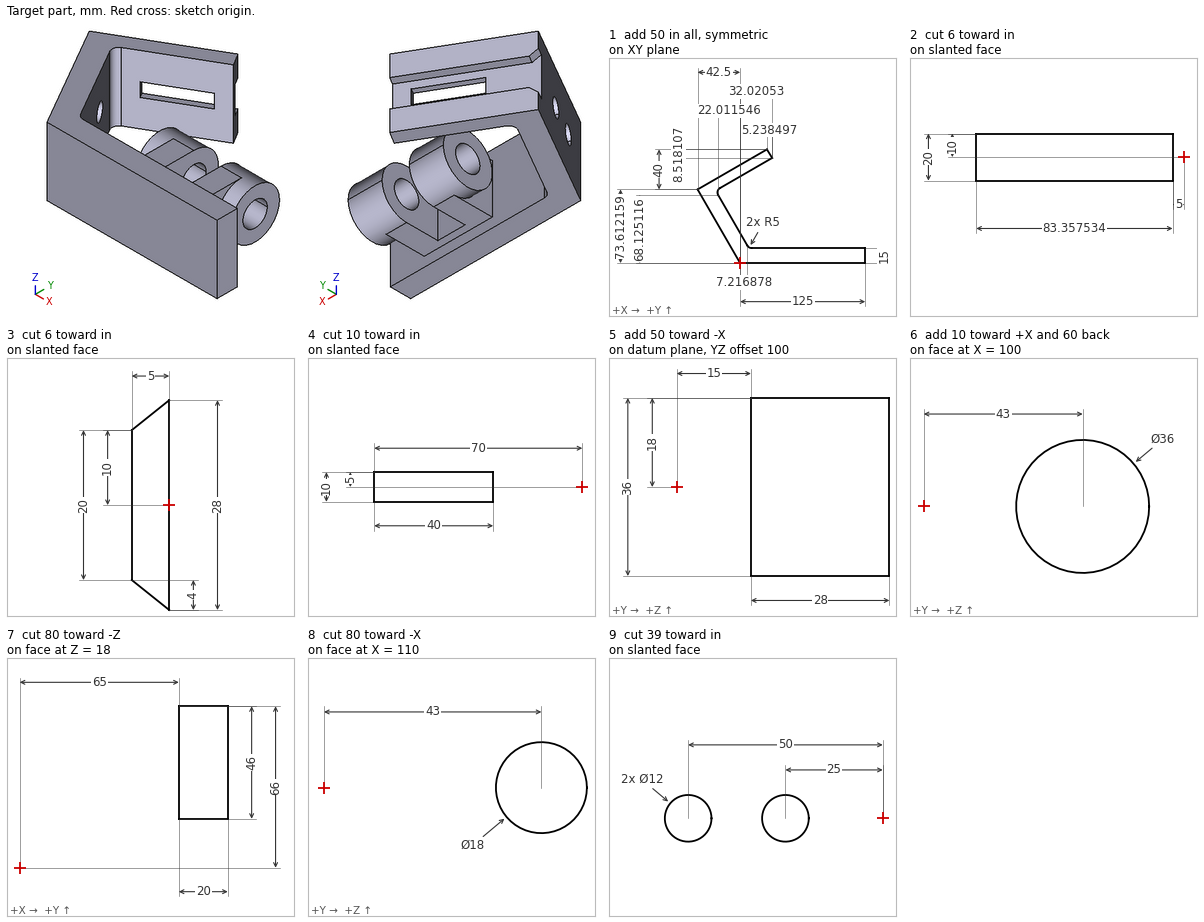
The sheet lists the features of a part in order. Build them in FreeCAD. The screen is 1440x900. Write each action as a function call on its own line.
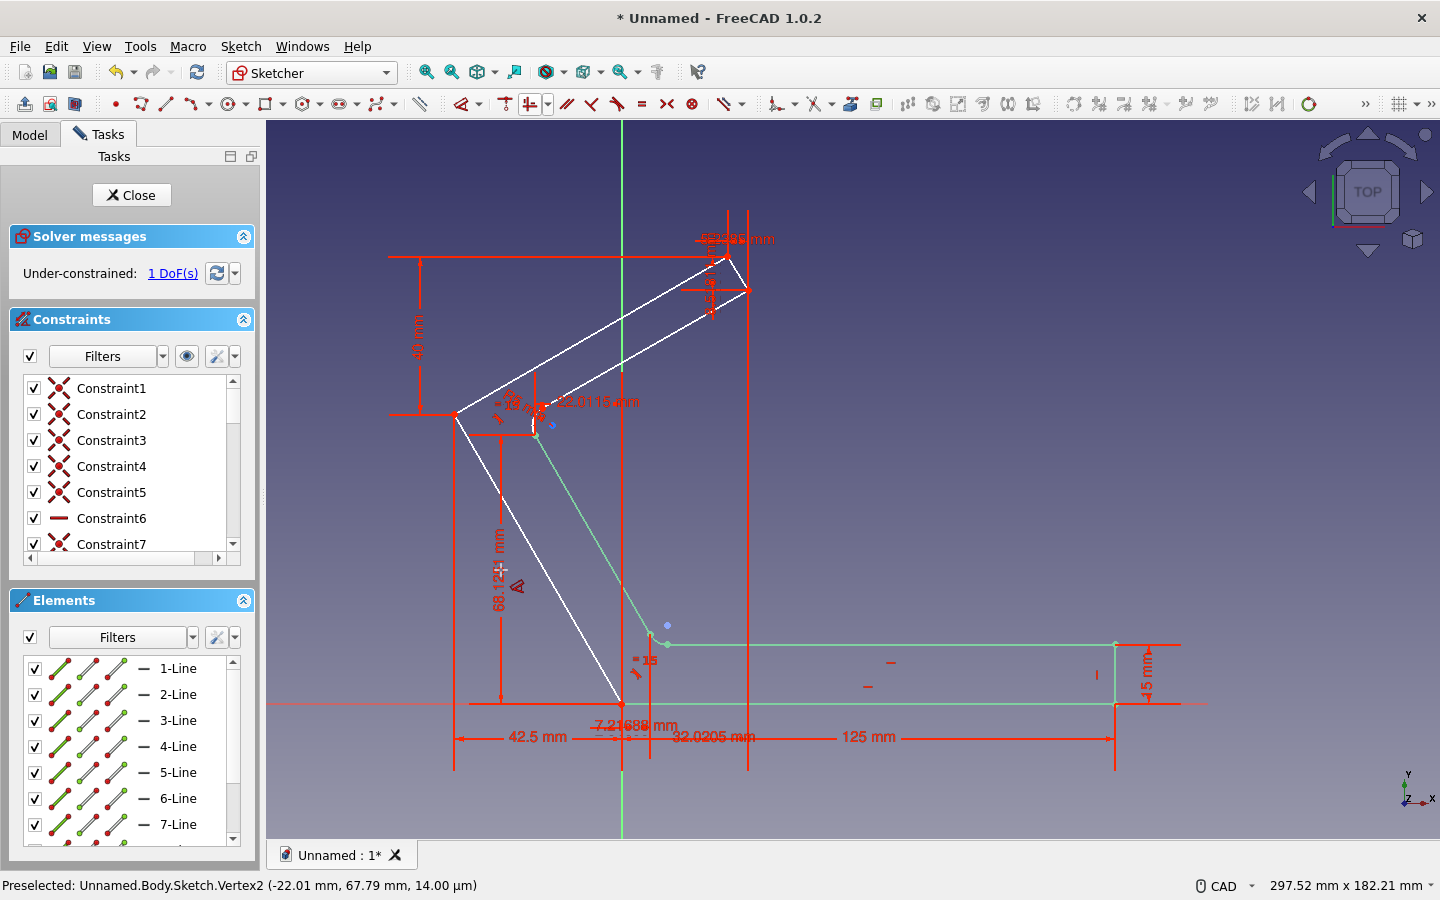
click(454, 415)
click(420, 559)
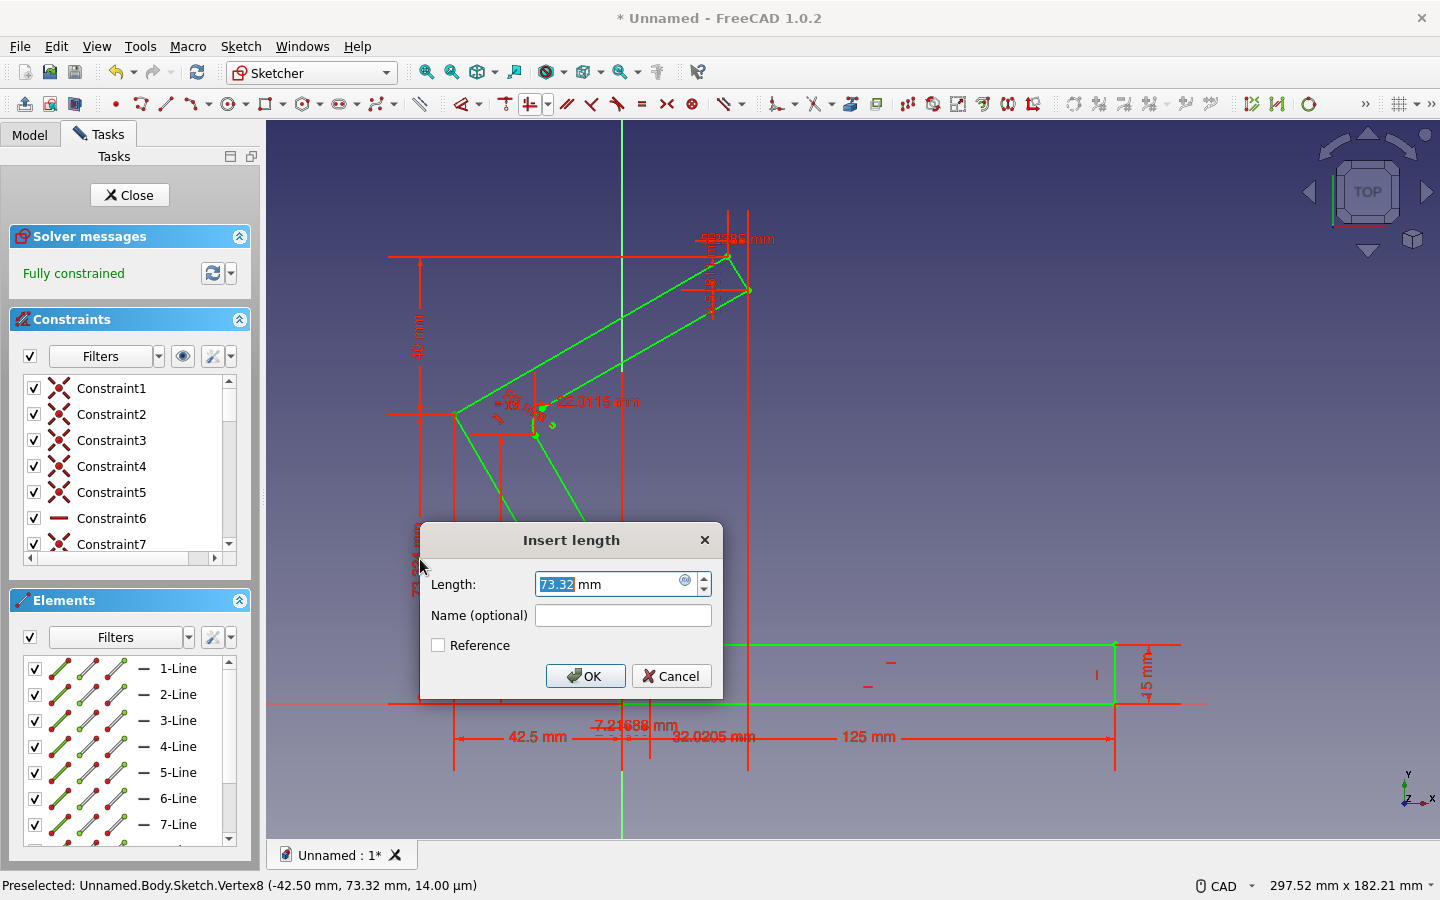
text(73.612159)
key(Return)
key(Escape)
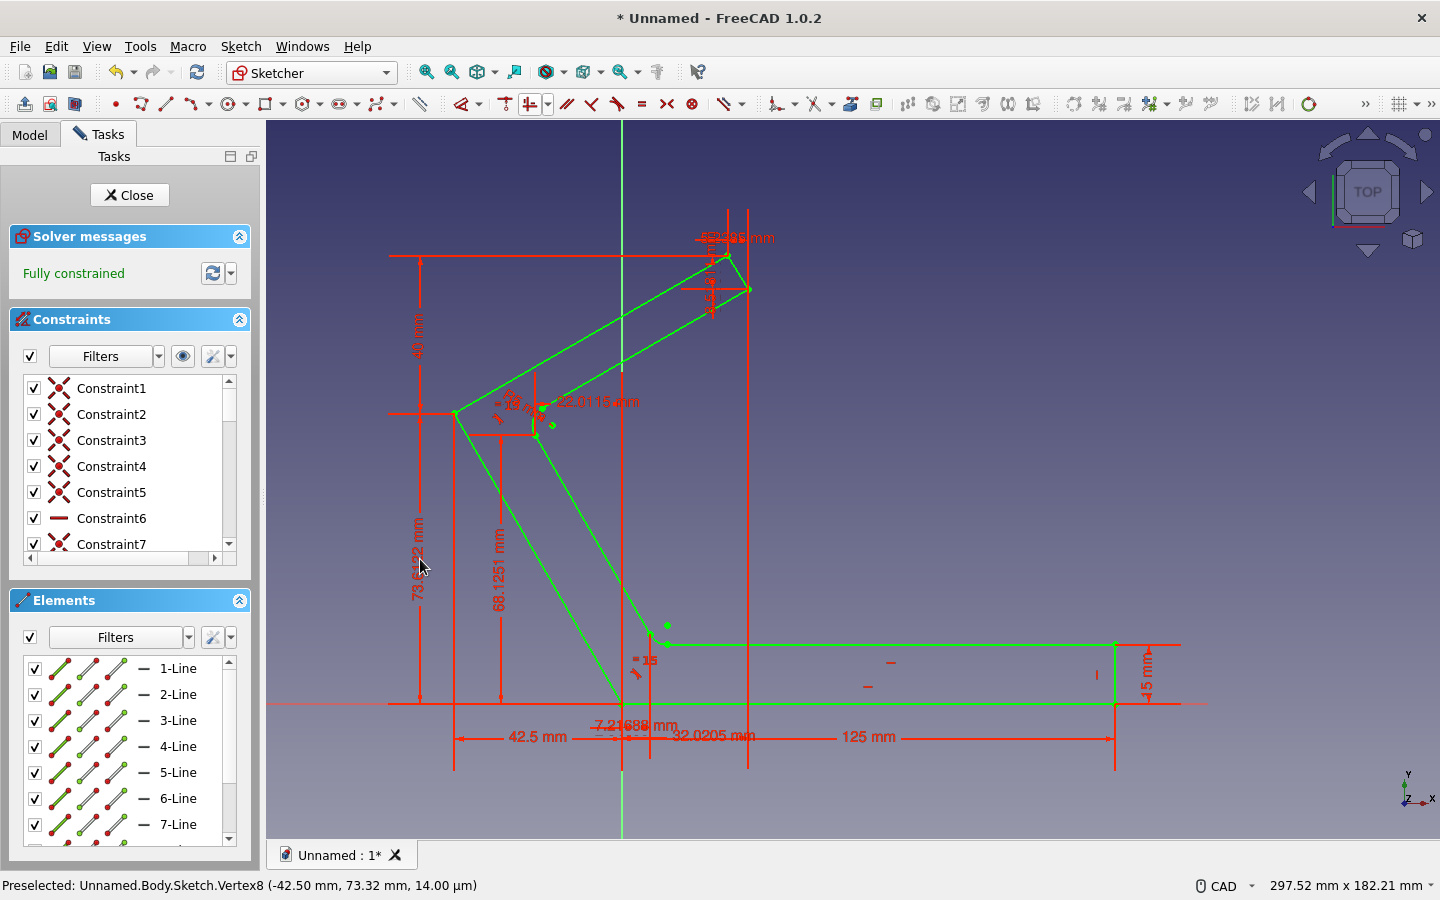
click(130, 195)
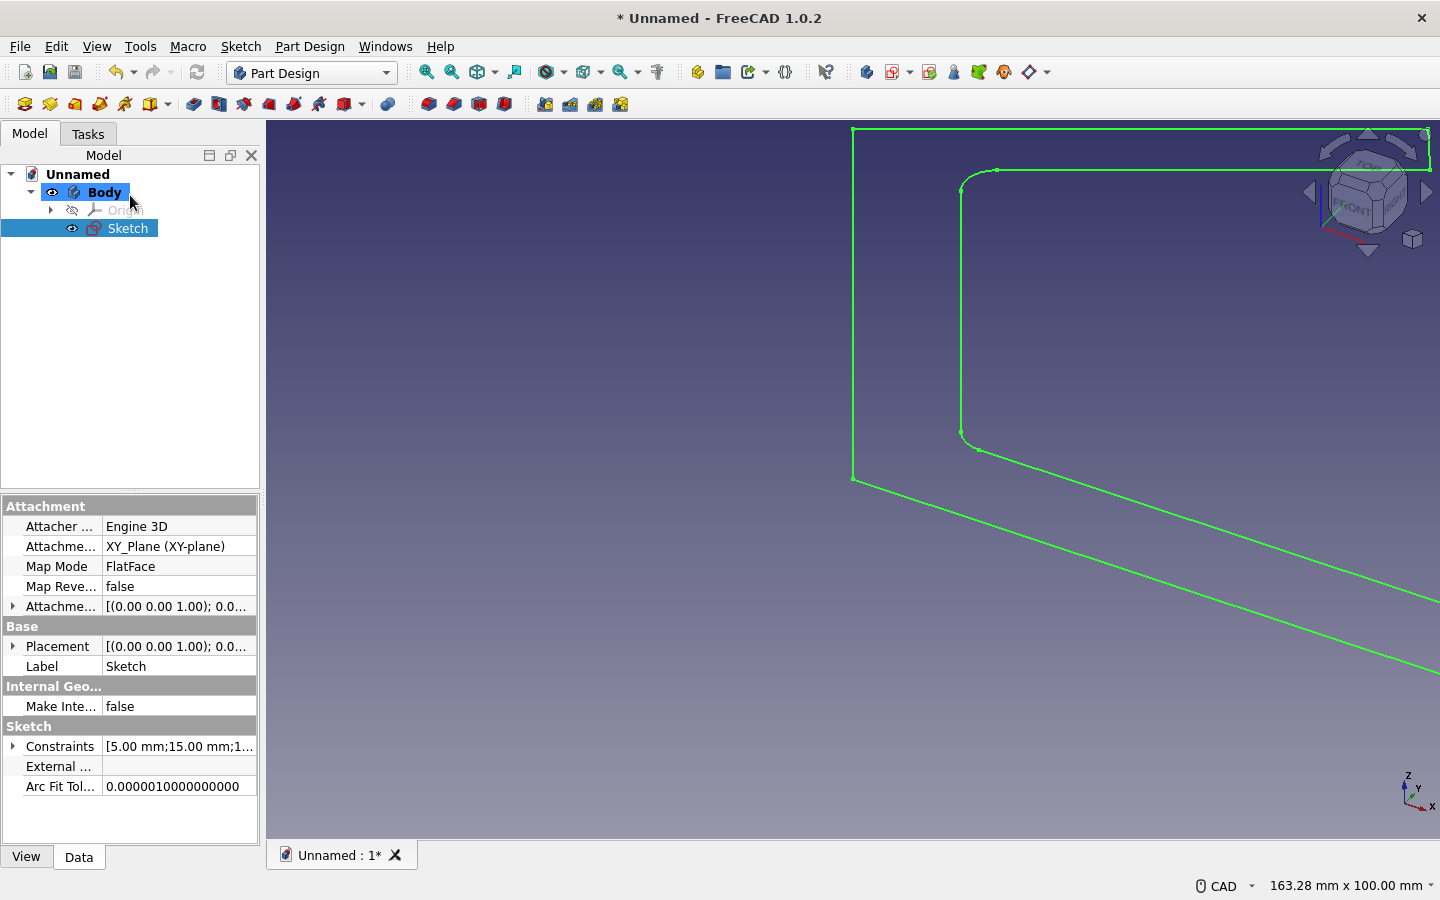
click(25, 104)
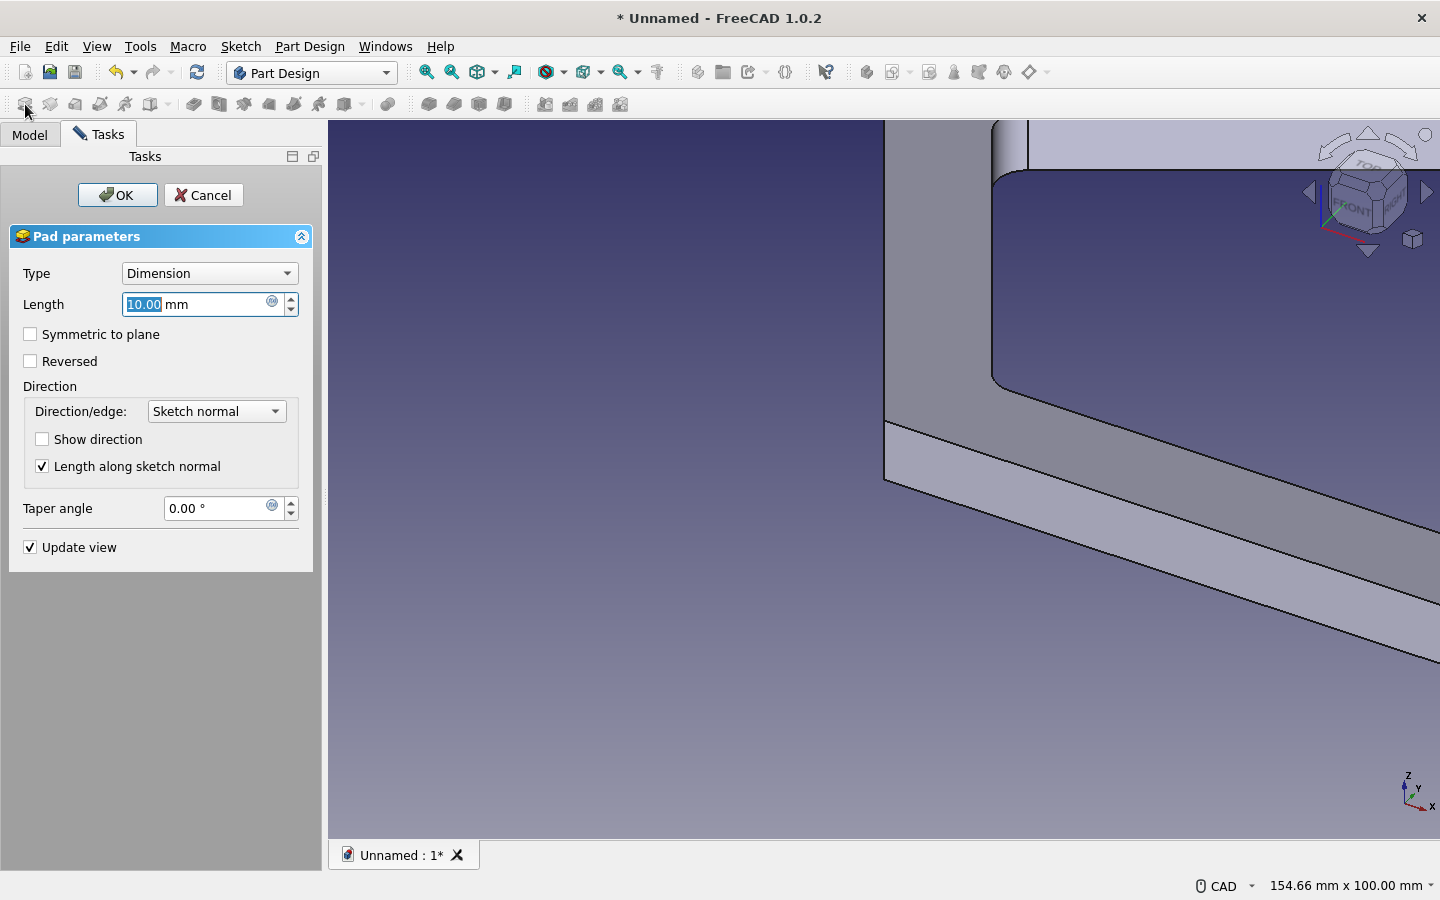
text(50)
key(Tab)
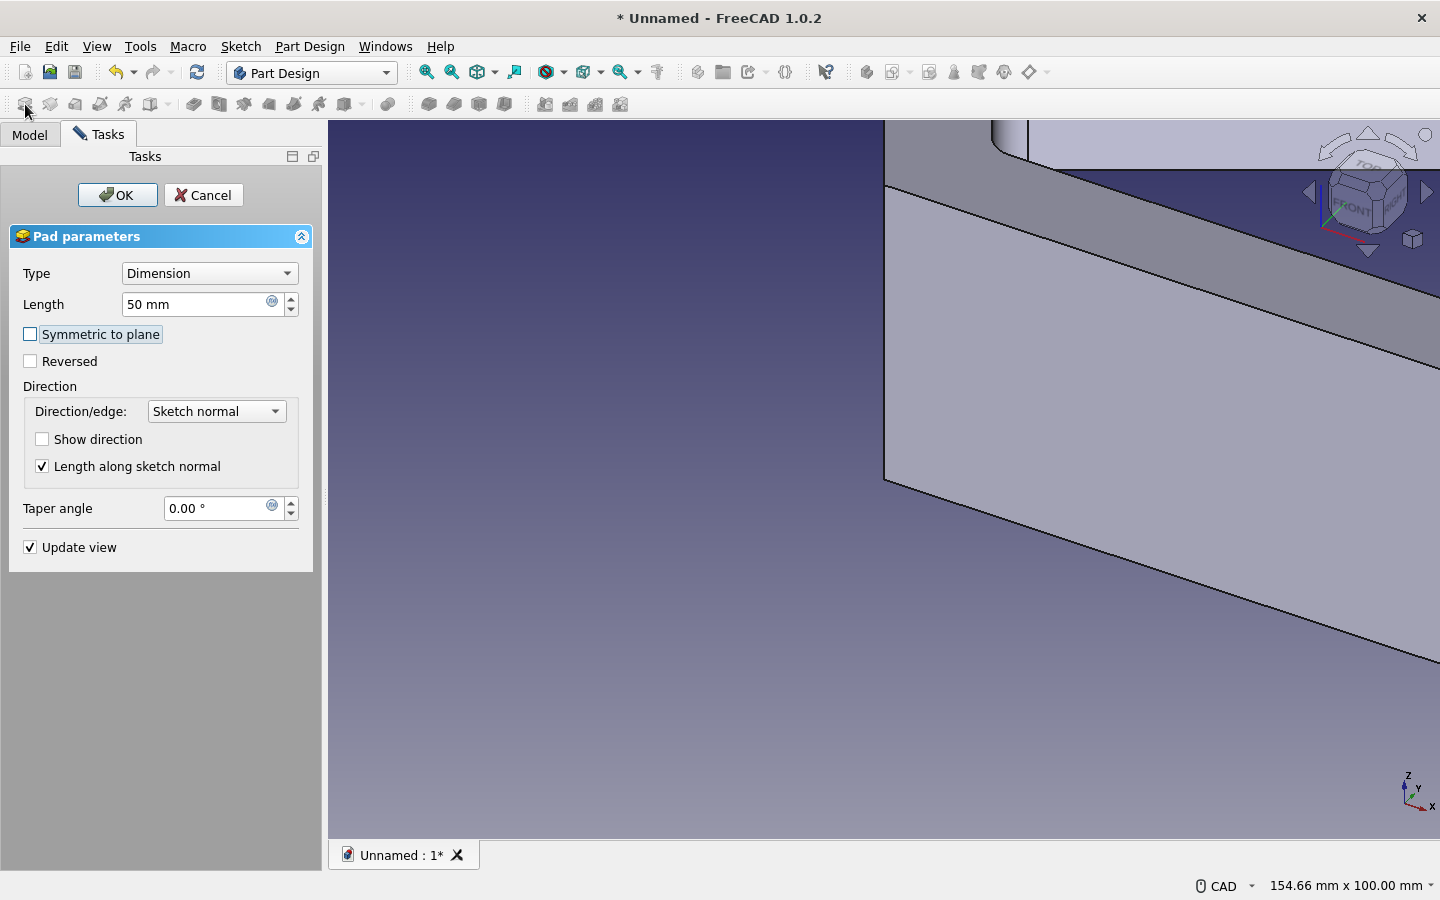
click(31, 334)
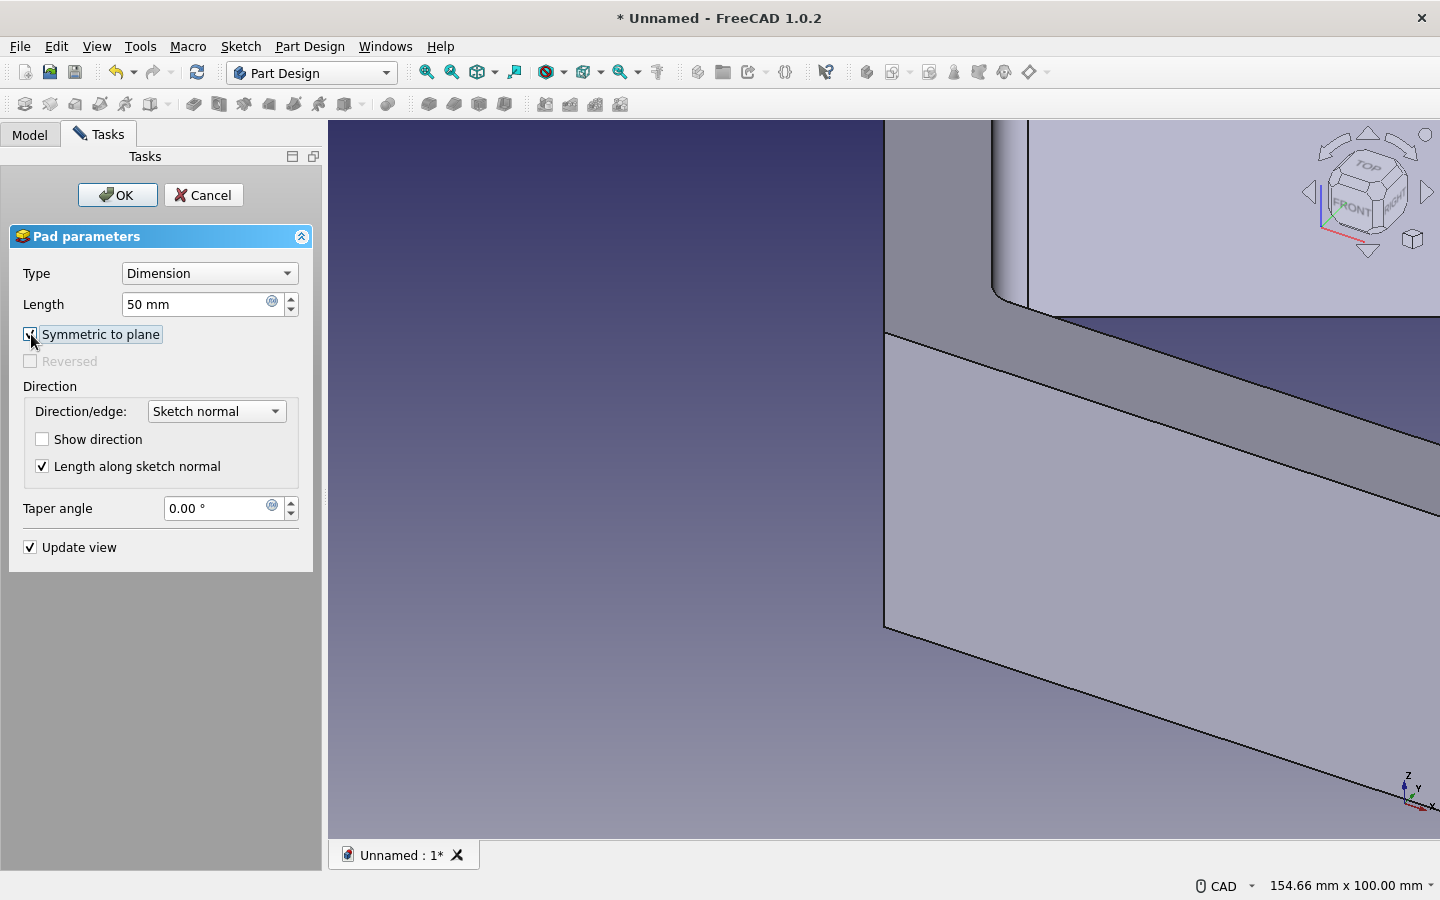
click(118, 195)